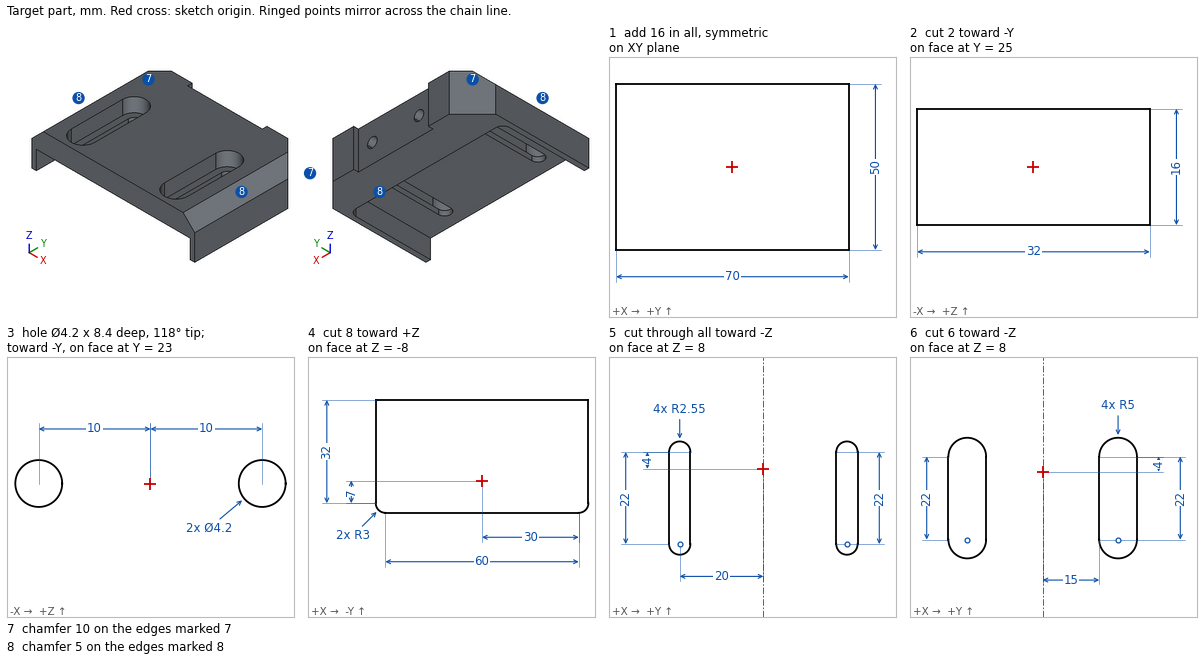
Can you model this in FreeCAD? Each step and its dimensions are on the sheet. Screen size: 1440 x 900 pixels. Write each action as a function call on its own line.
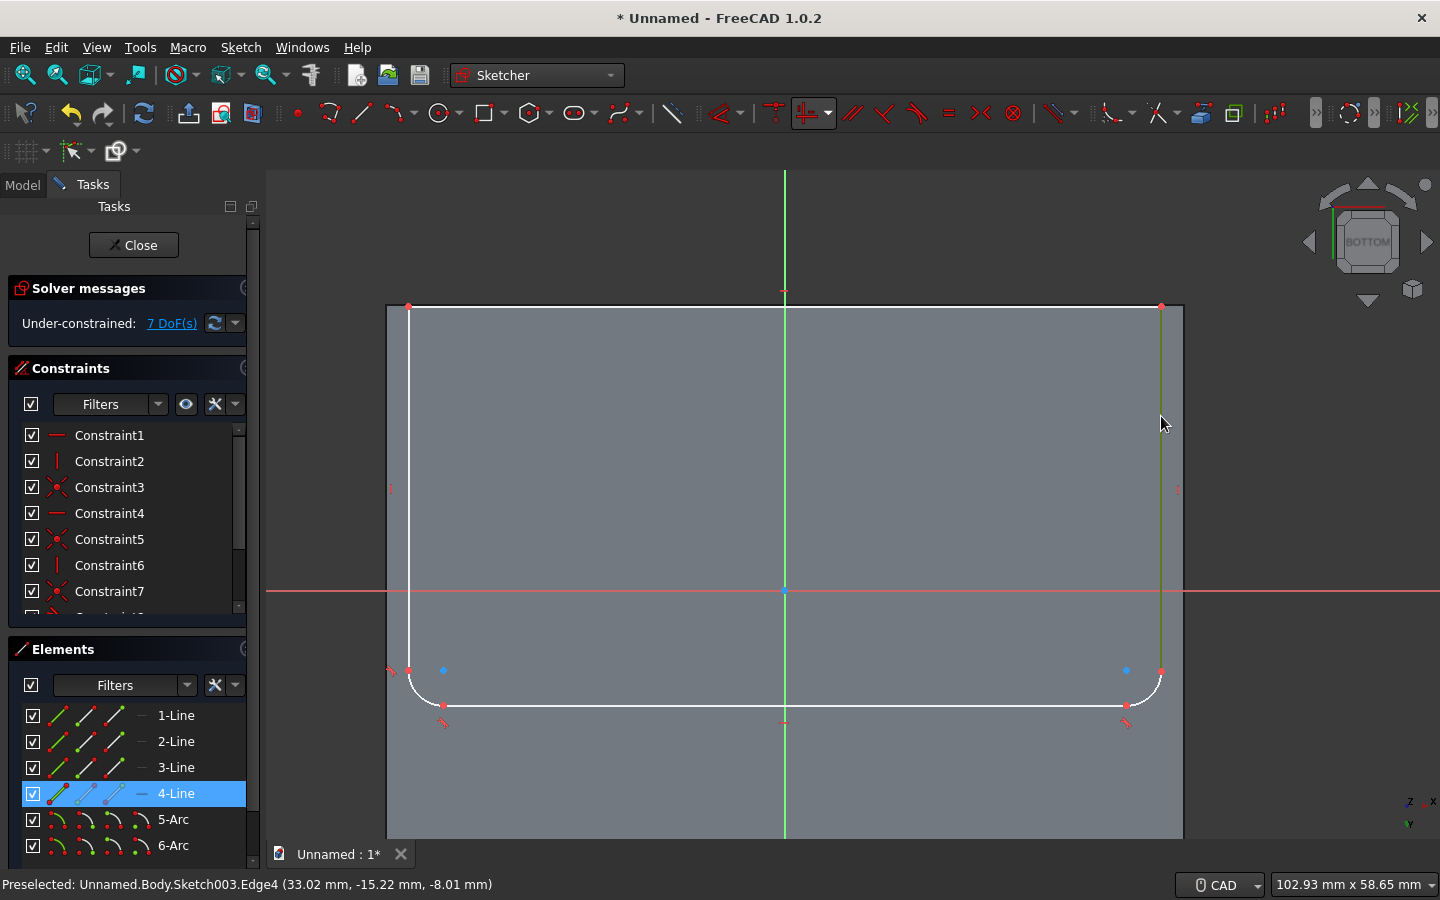
click(1142, 702)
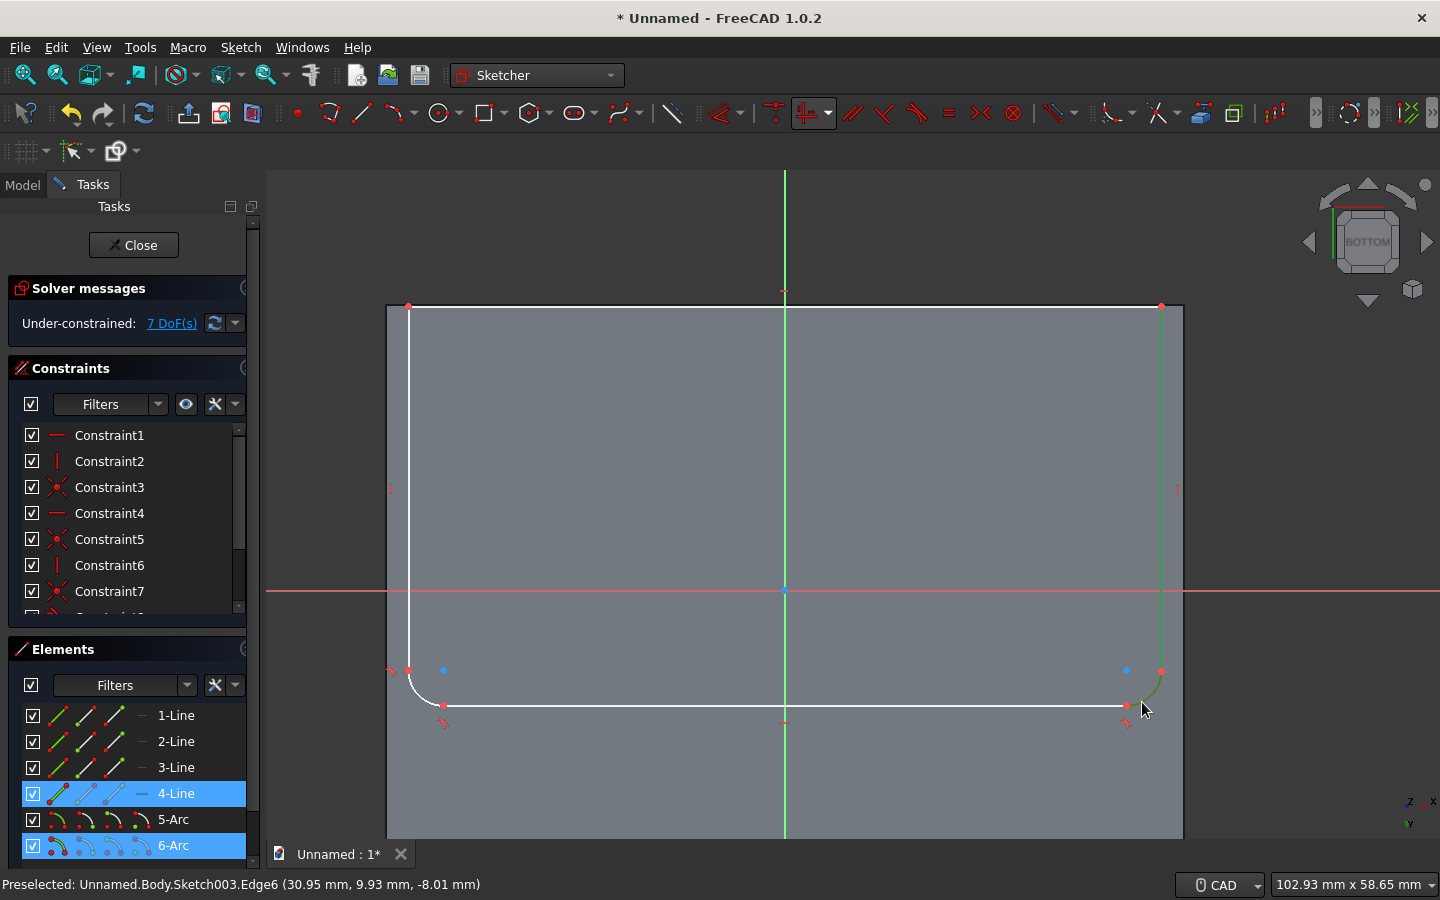
click(918, 114)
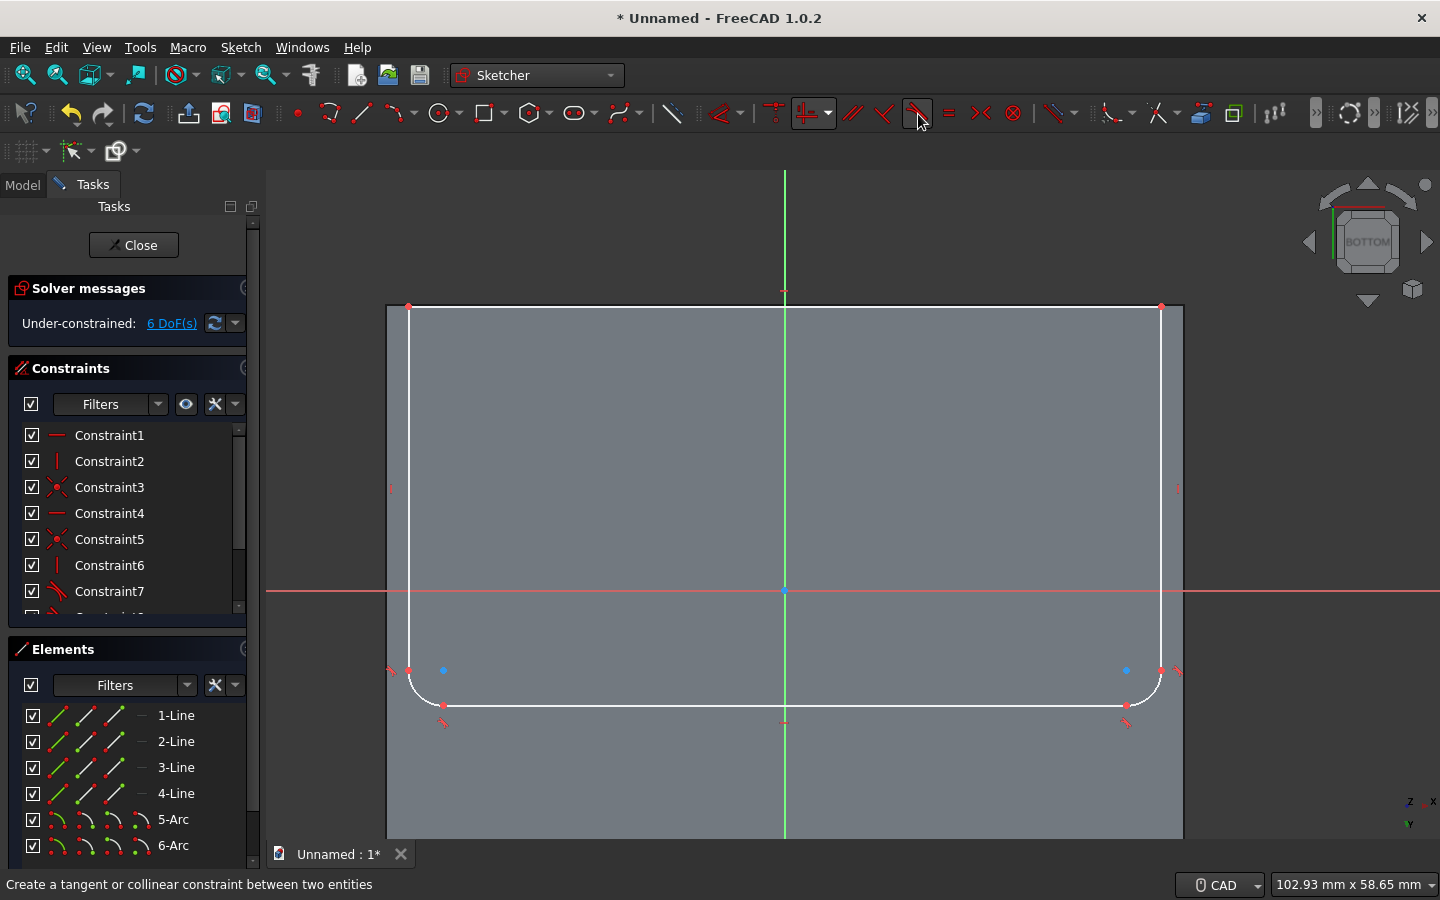
click(412, 687)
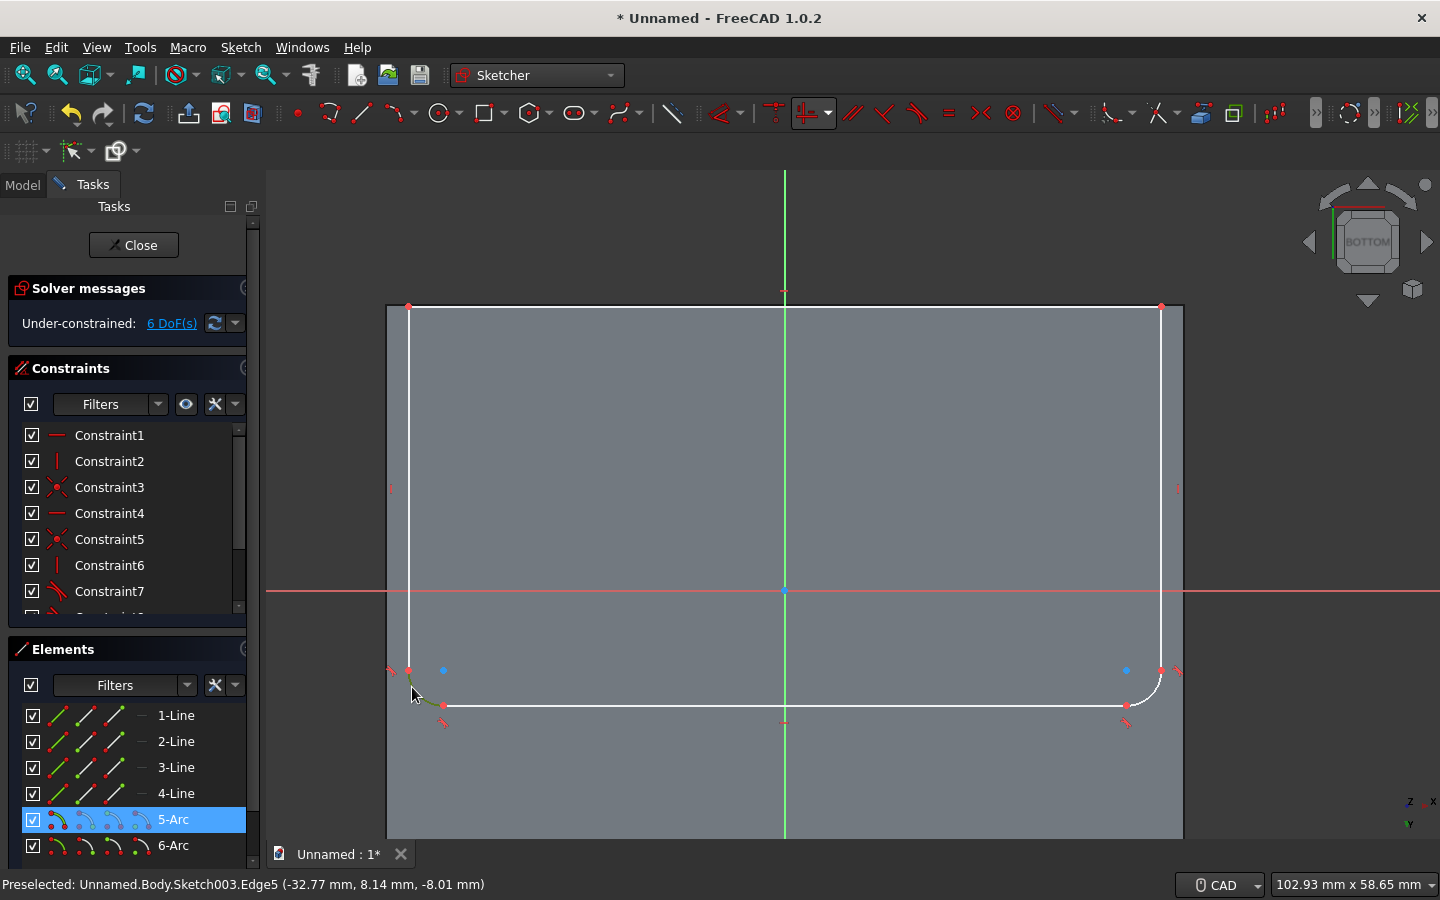
click(1142, 702)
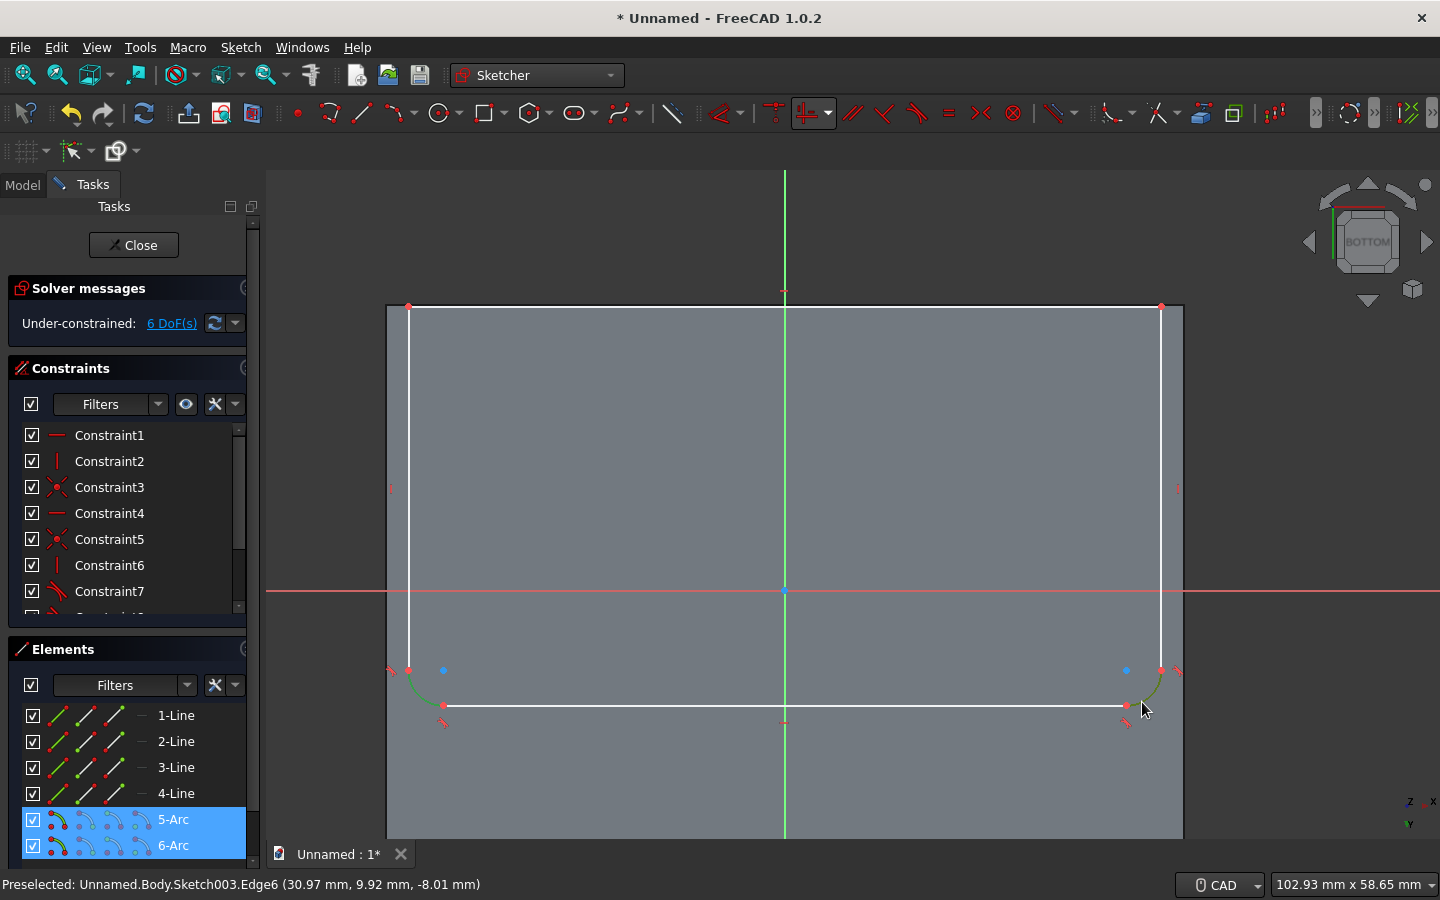
click(950, 114)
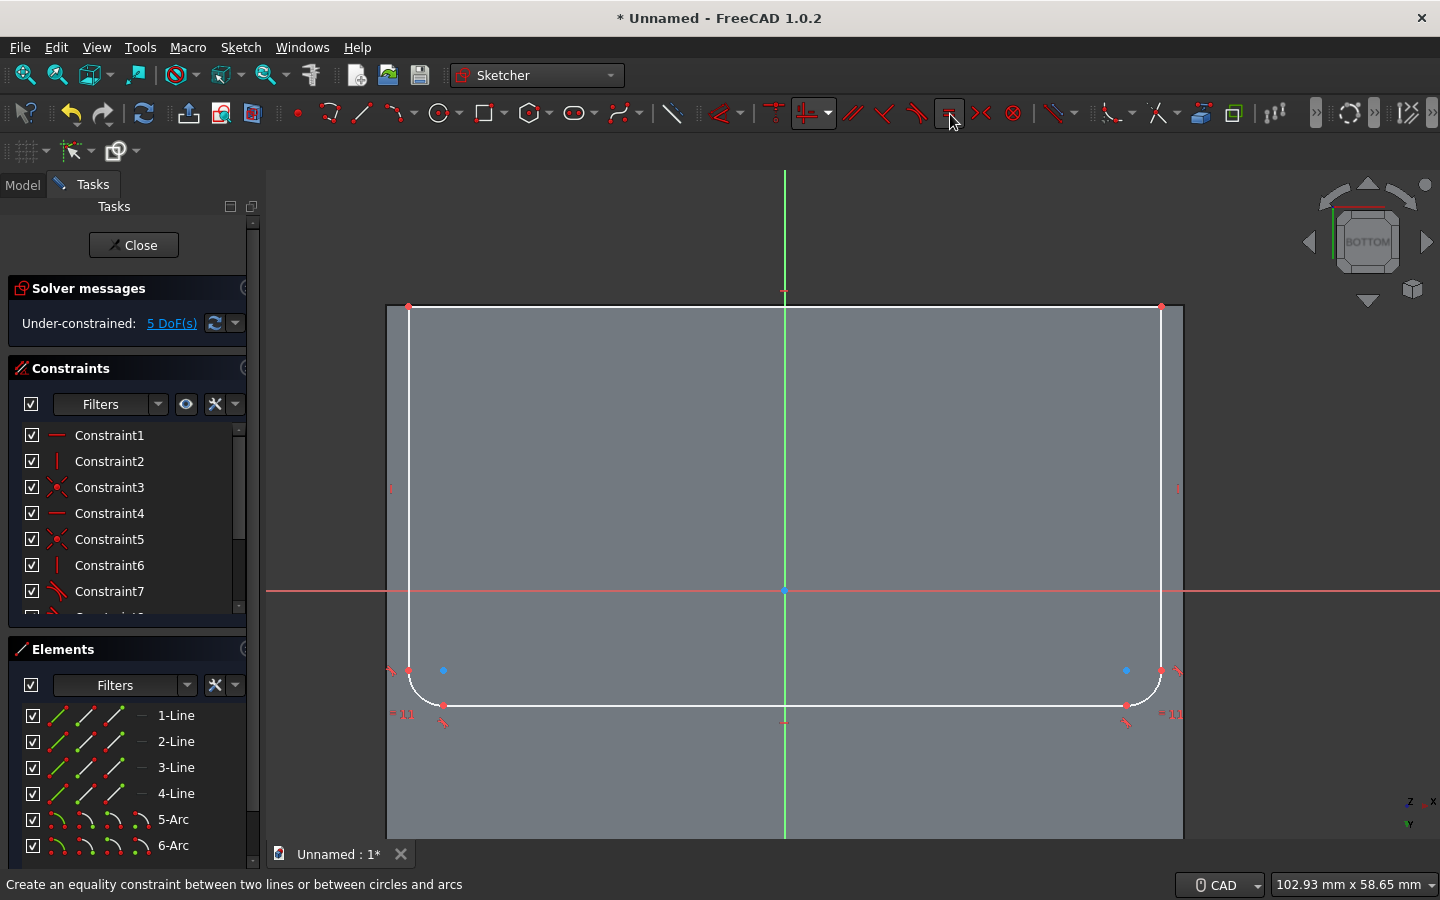
click(720, 114)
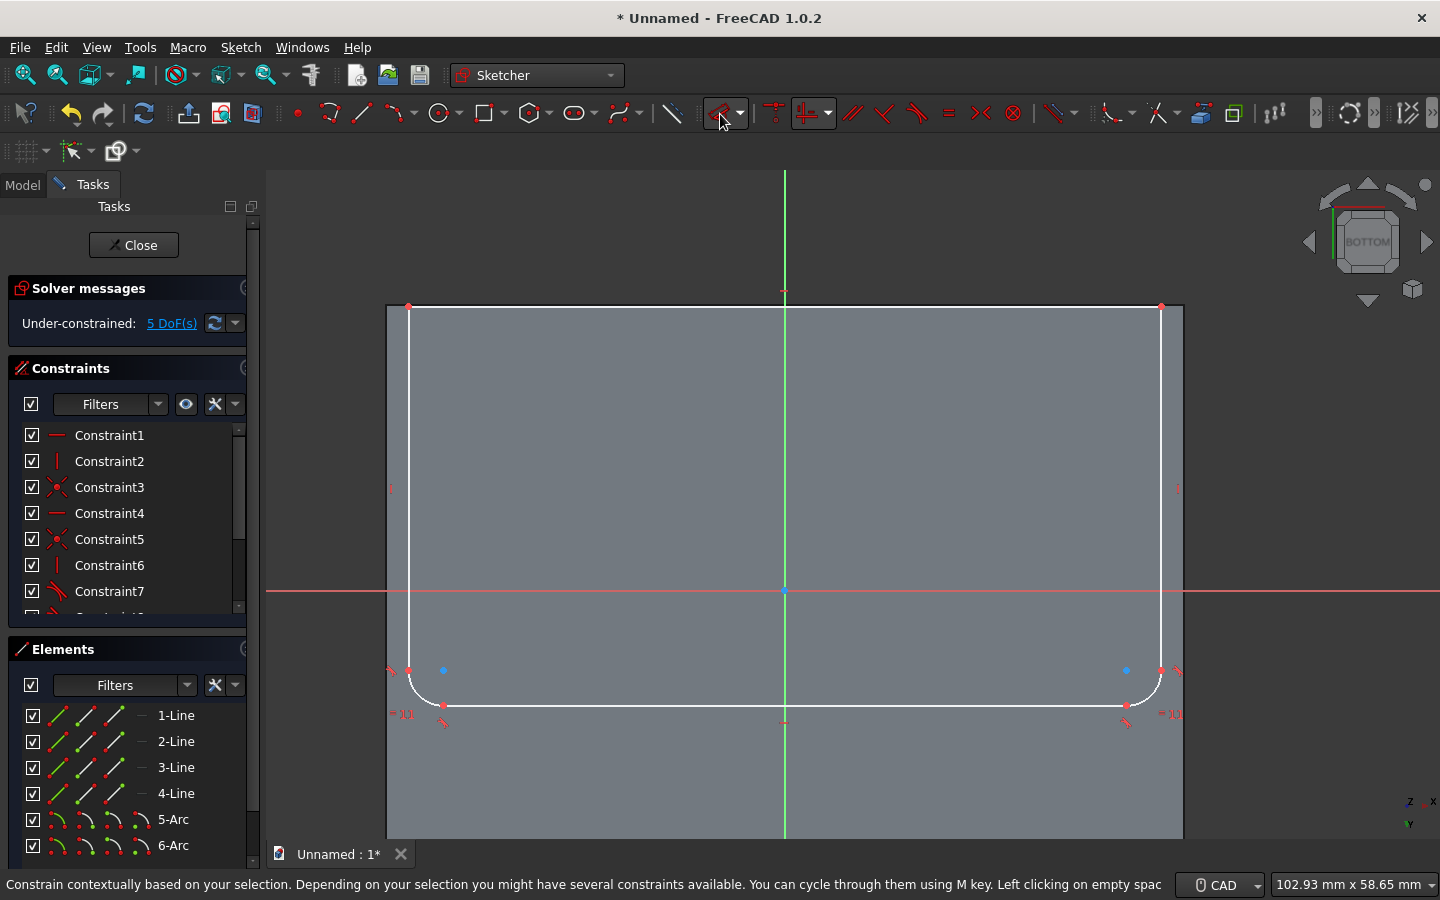
click(412, 687)
click(384, 702)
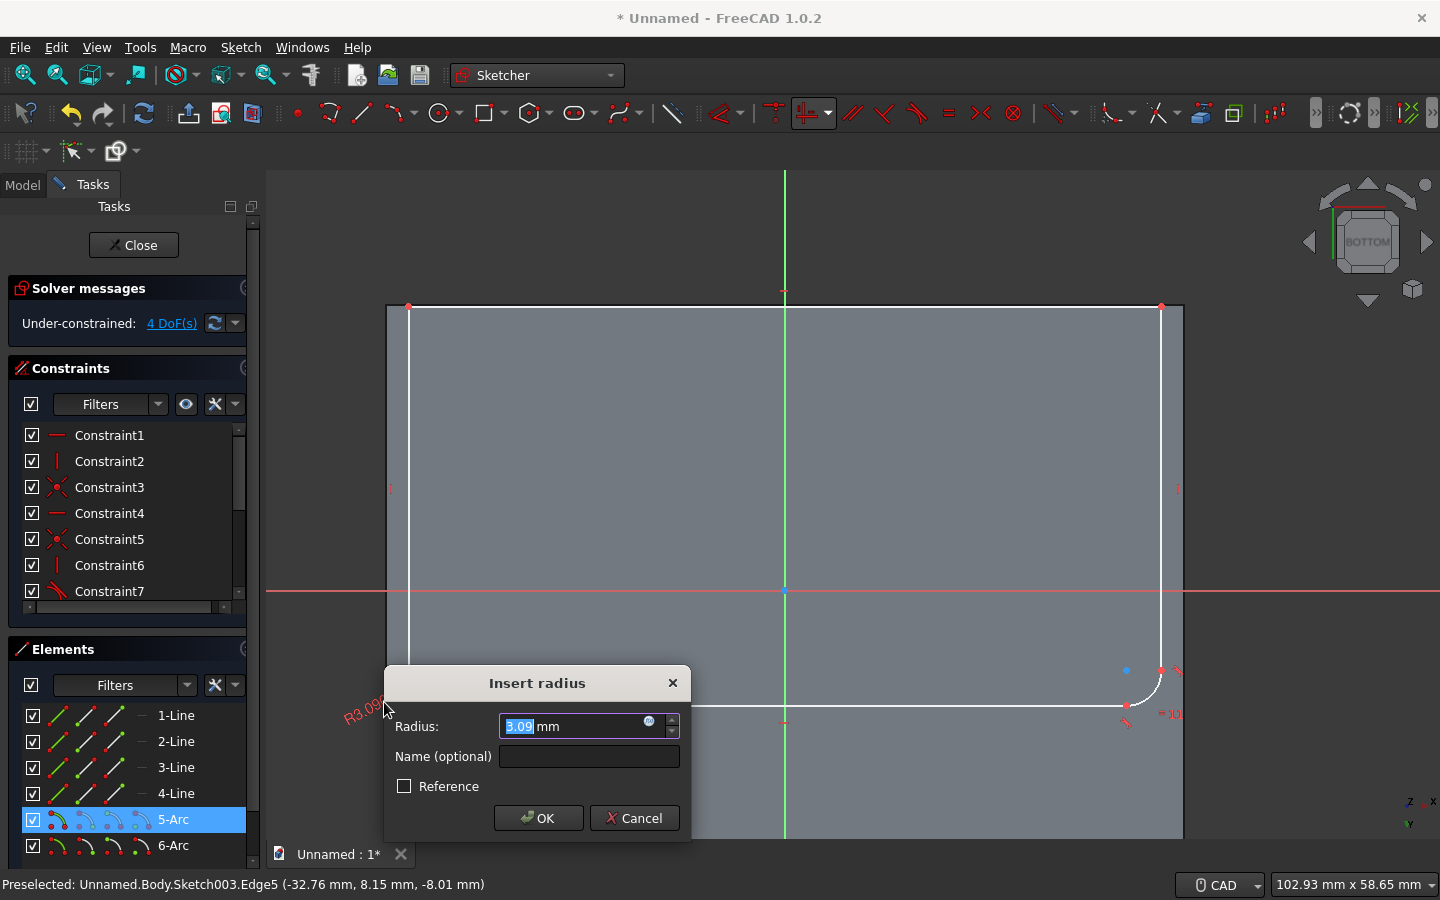
text(3)
key(Return)